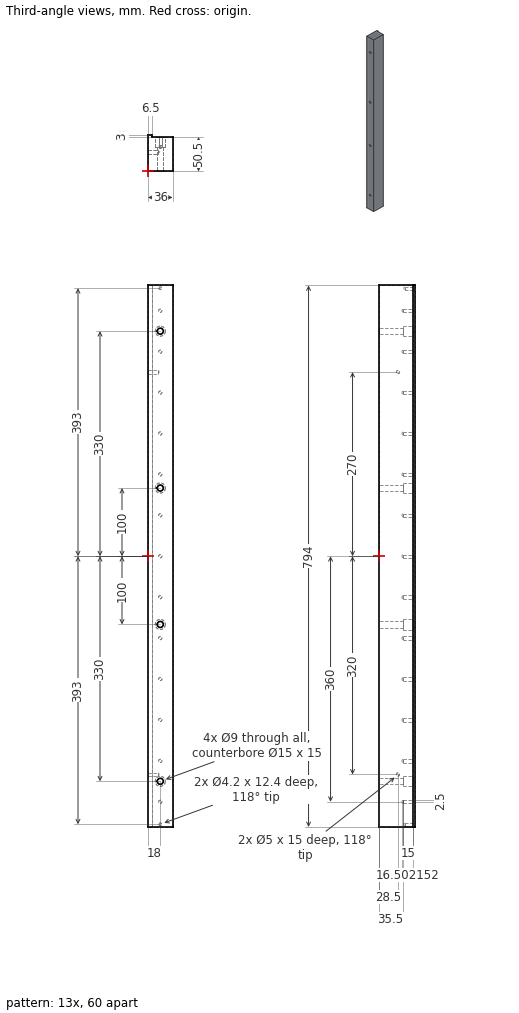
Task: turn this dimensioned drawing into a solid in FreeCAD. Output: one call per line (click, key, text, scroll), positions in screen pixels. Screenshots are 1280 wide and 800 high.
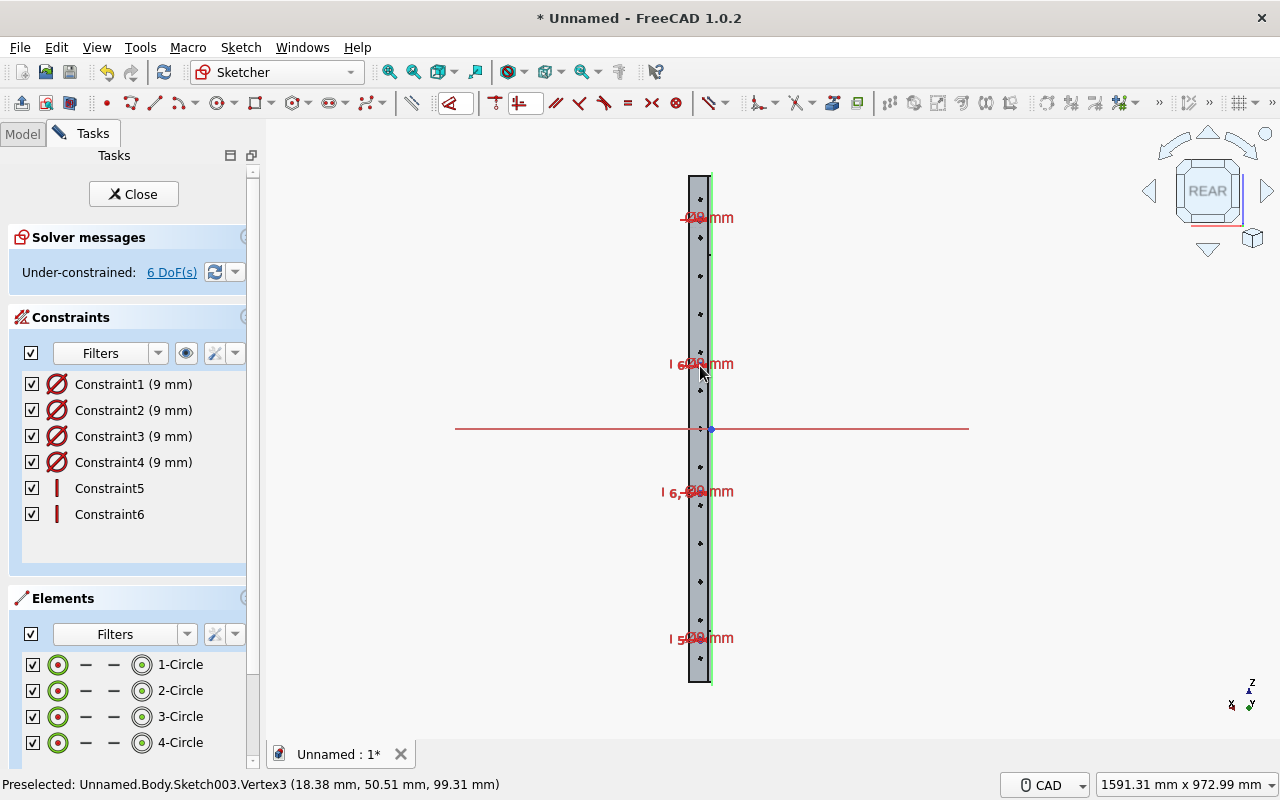
click(700, 366)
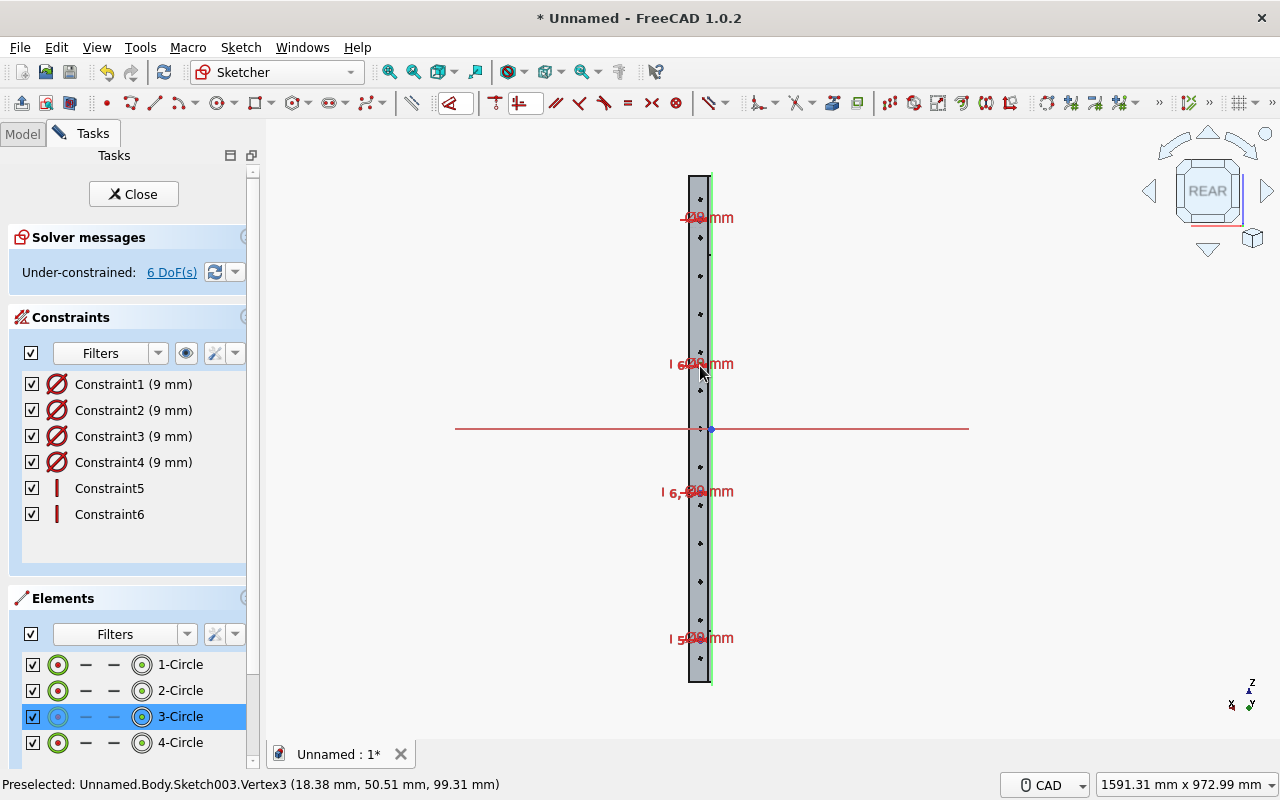
click(700, 220)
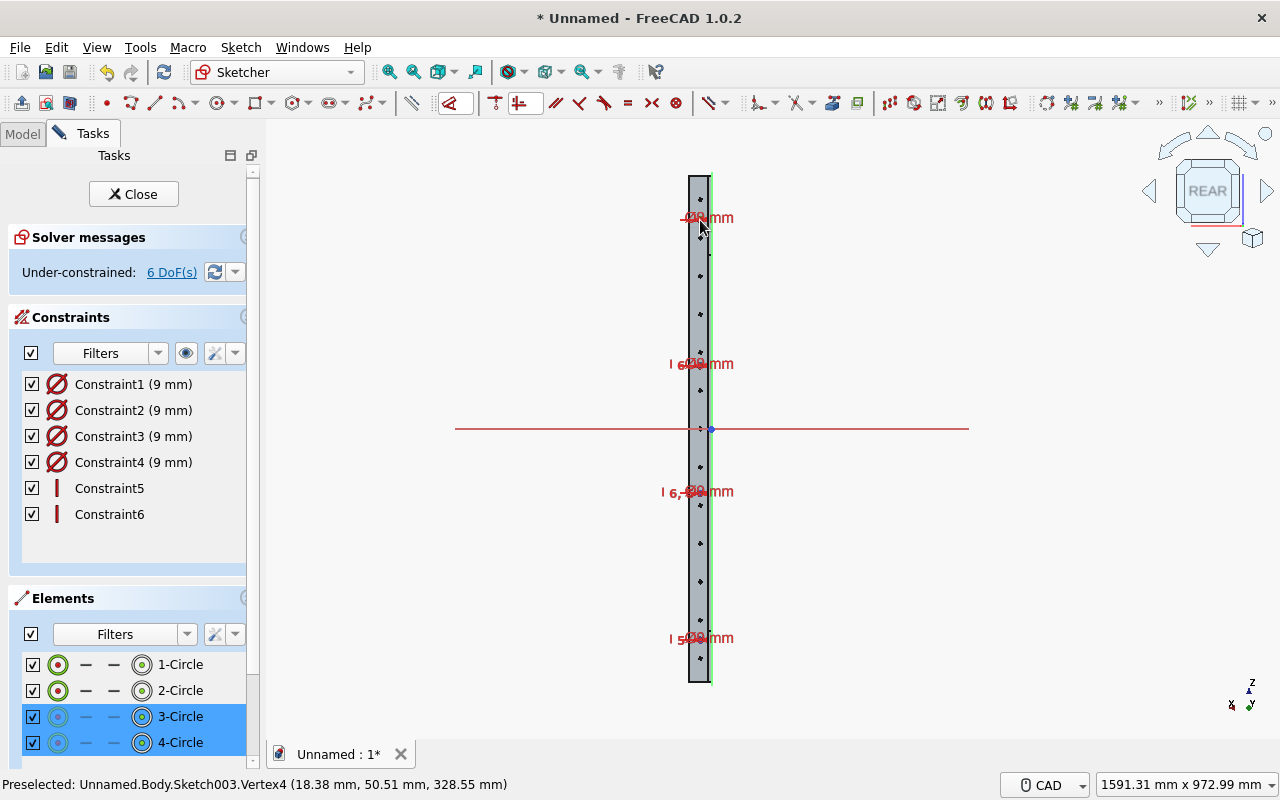
click(538, 104)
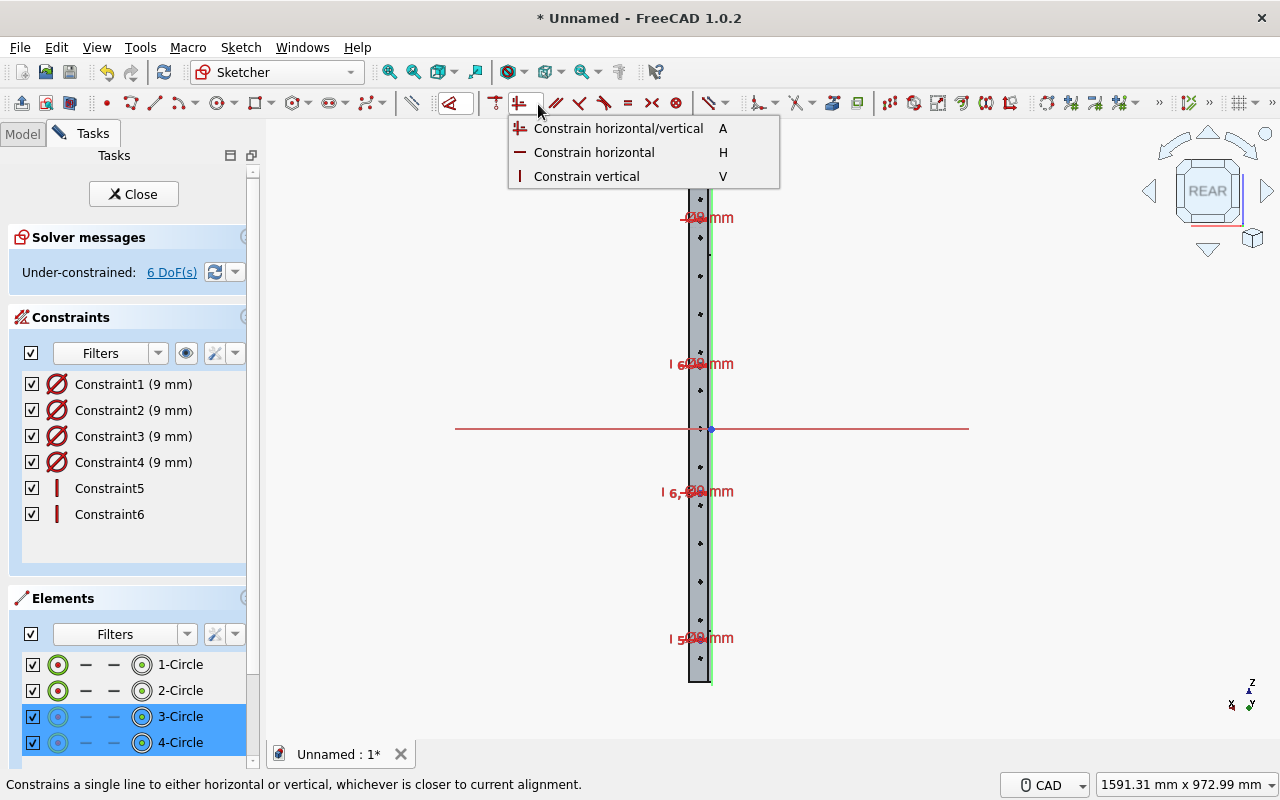
click(644, 176)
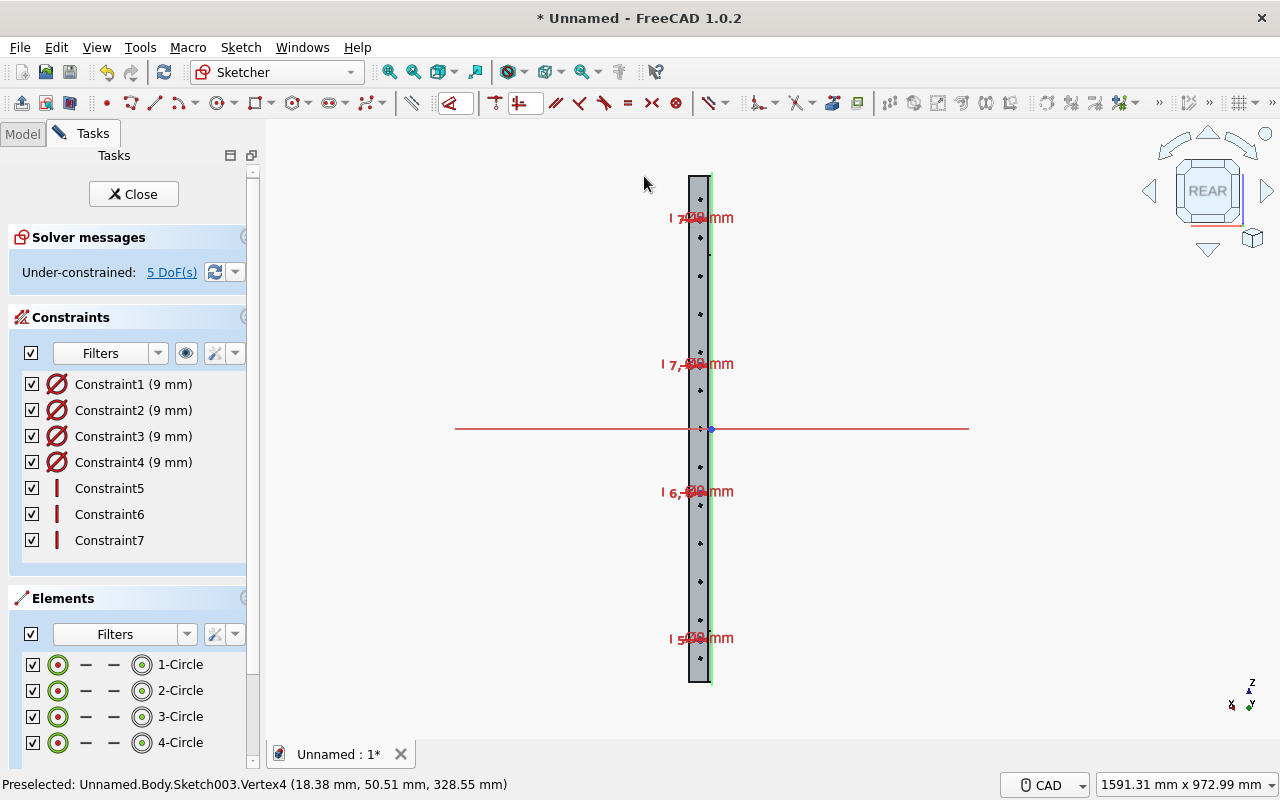
scroll(700, 640, up, 7)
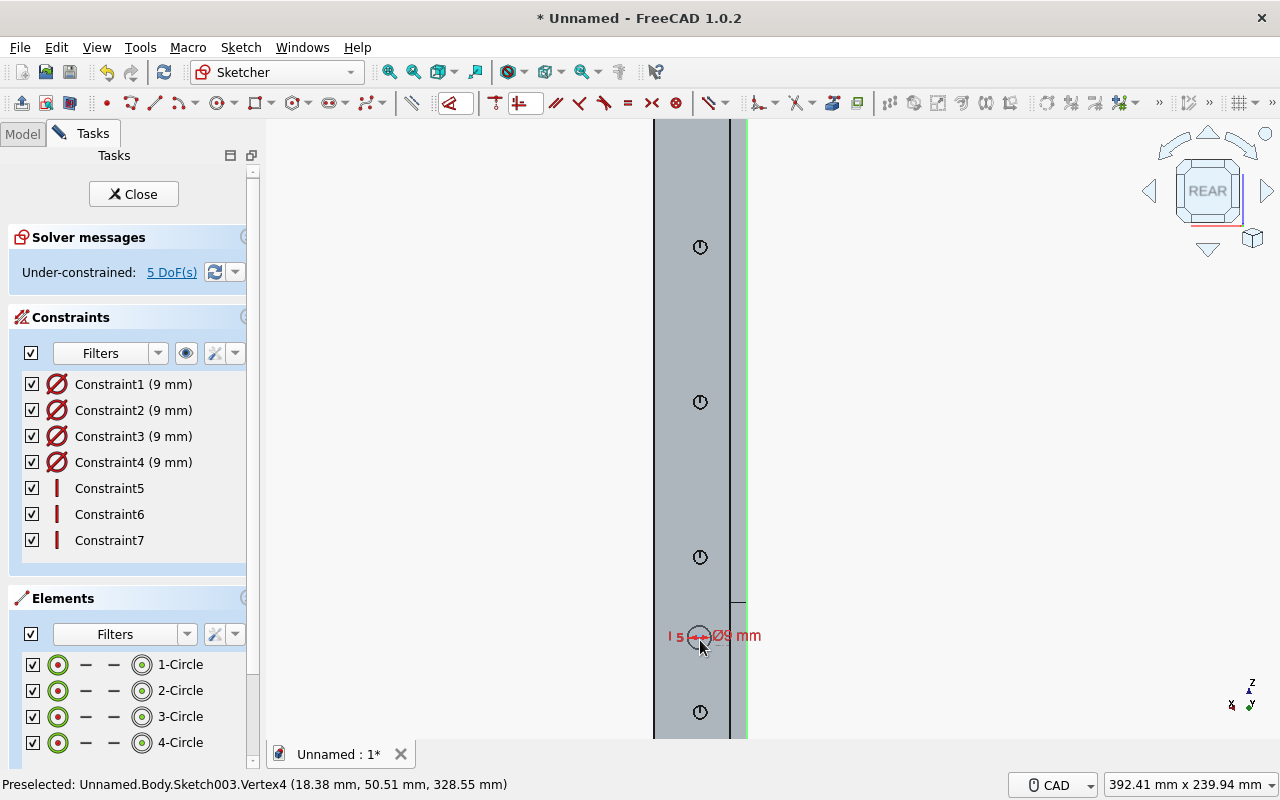
click(699, 638)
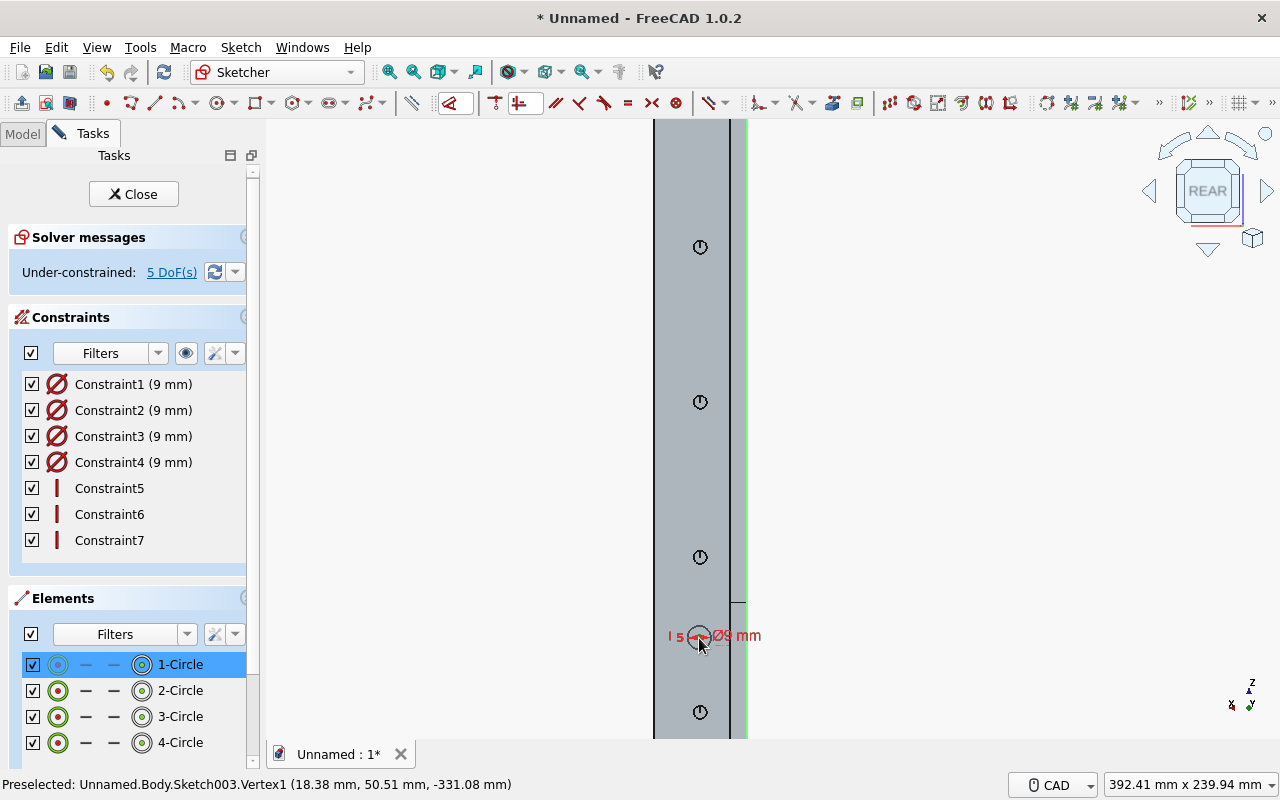
key(l)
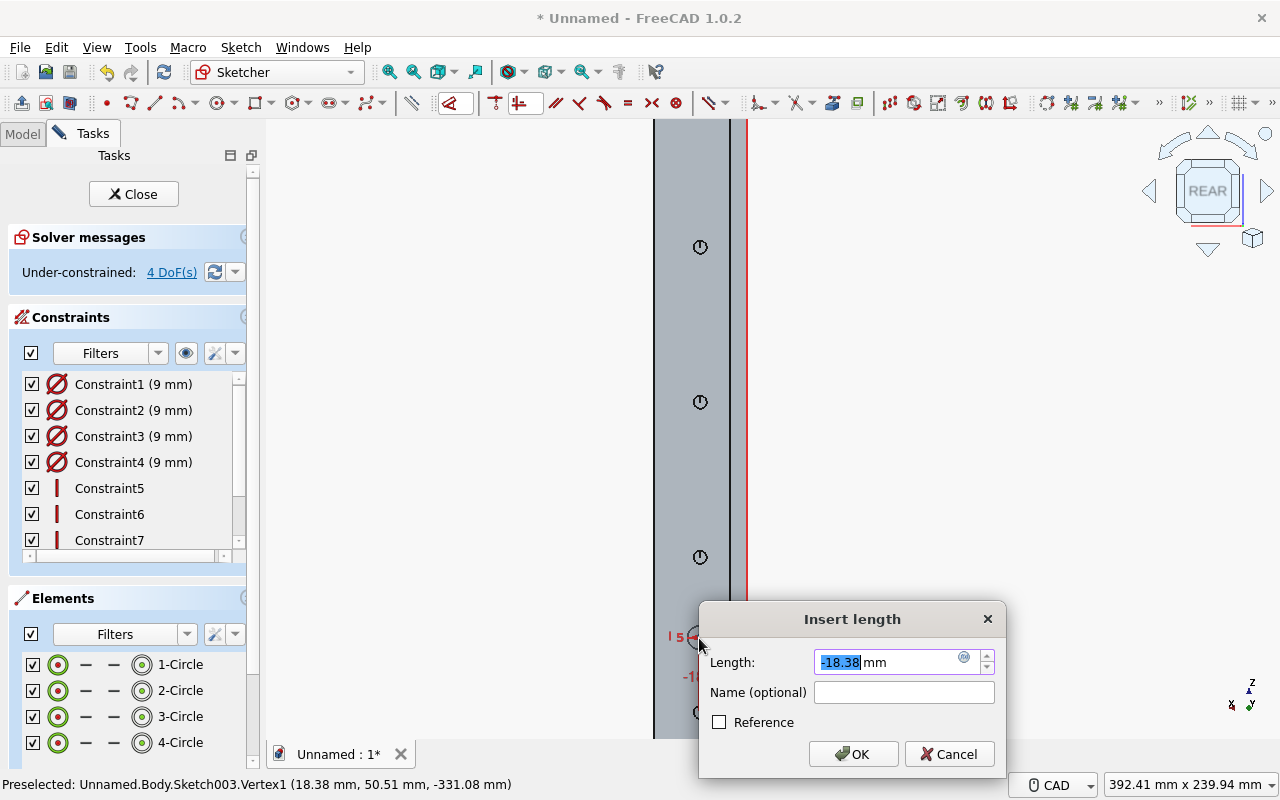
text(-18)
key(Return)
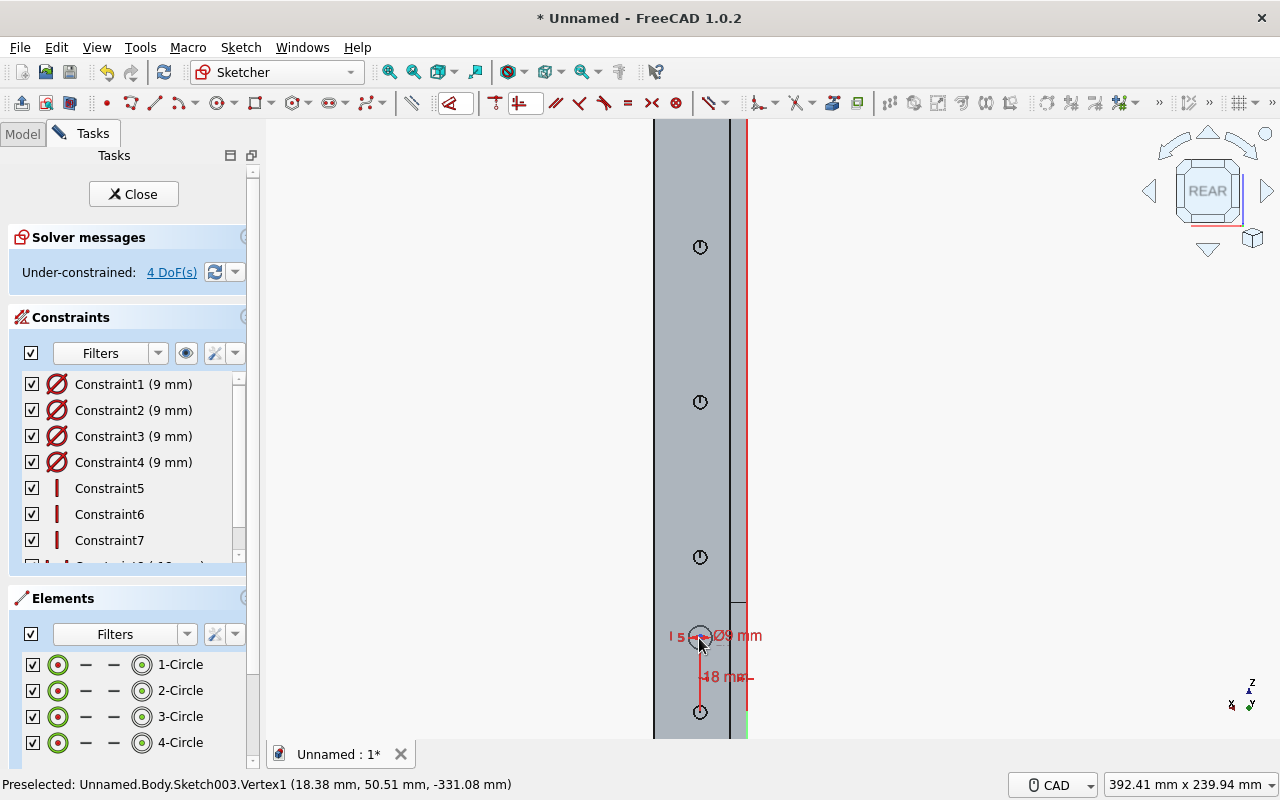
scroll(700, 641, down, 7)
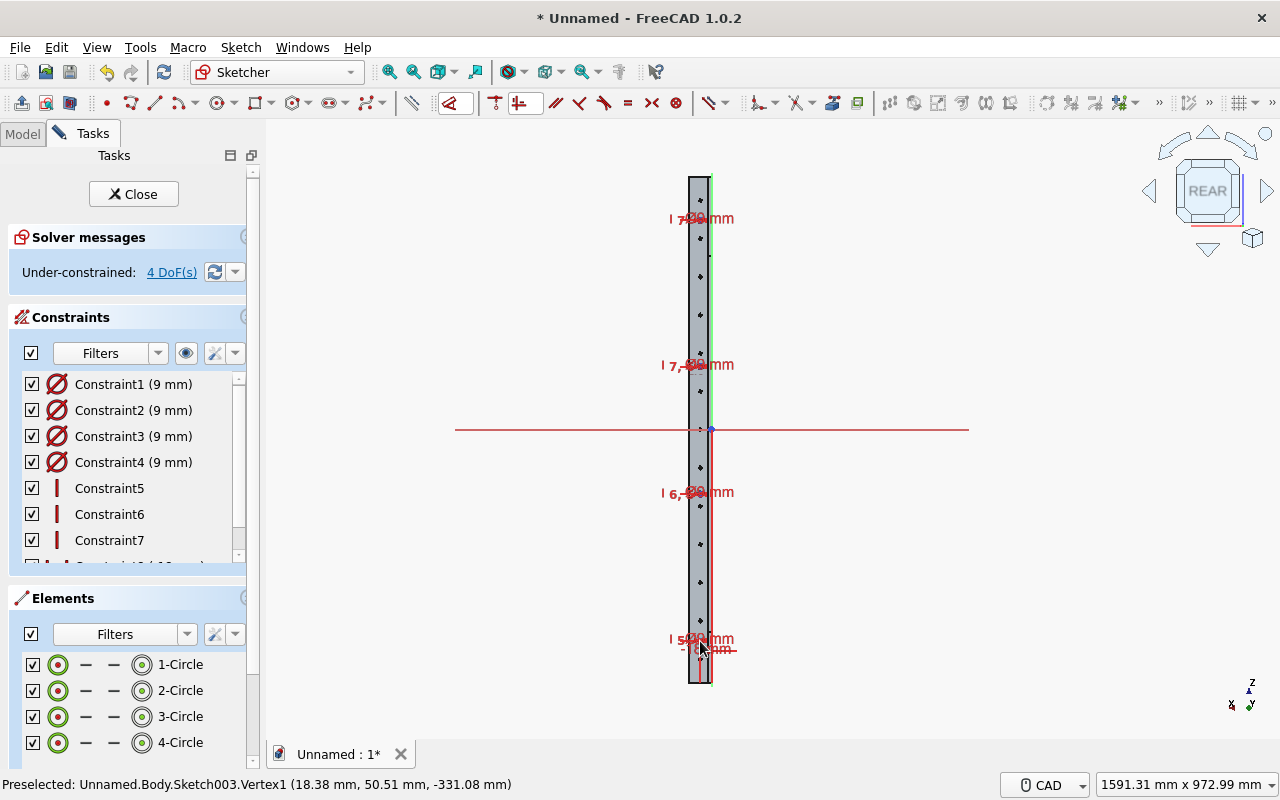
click(700, 641)